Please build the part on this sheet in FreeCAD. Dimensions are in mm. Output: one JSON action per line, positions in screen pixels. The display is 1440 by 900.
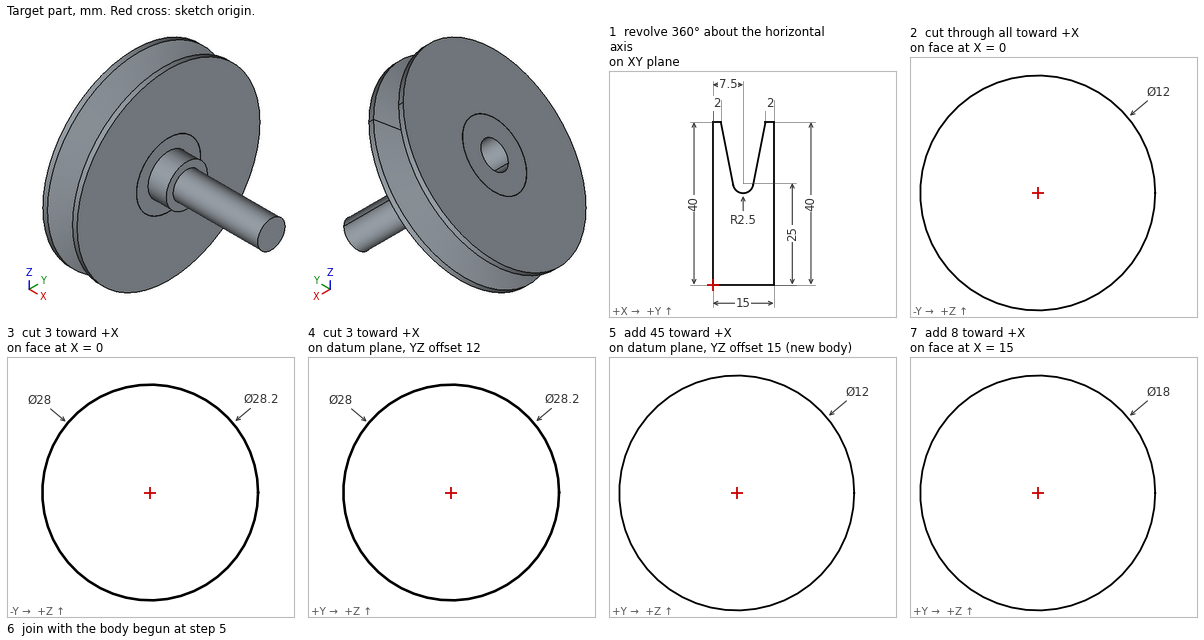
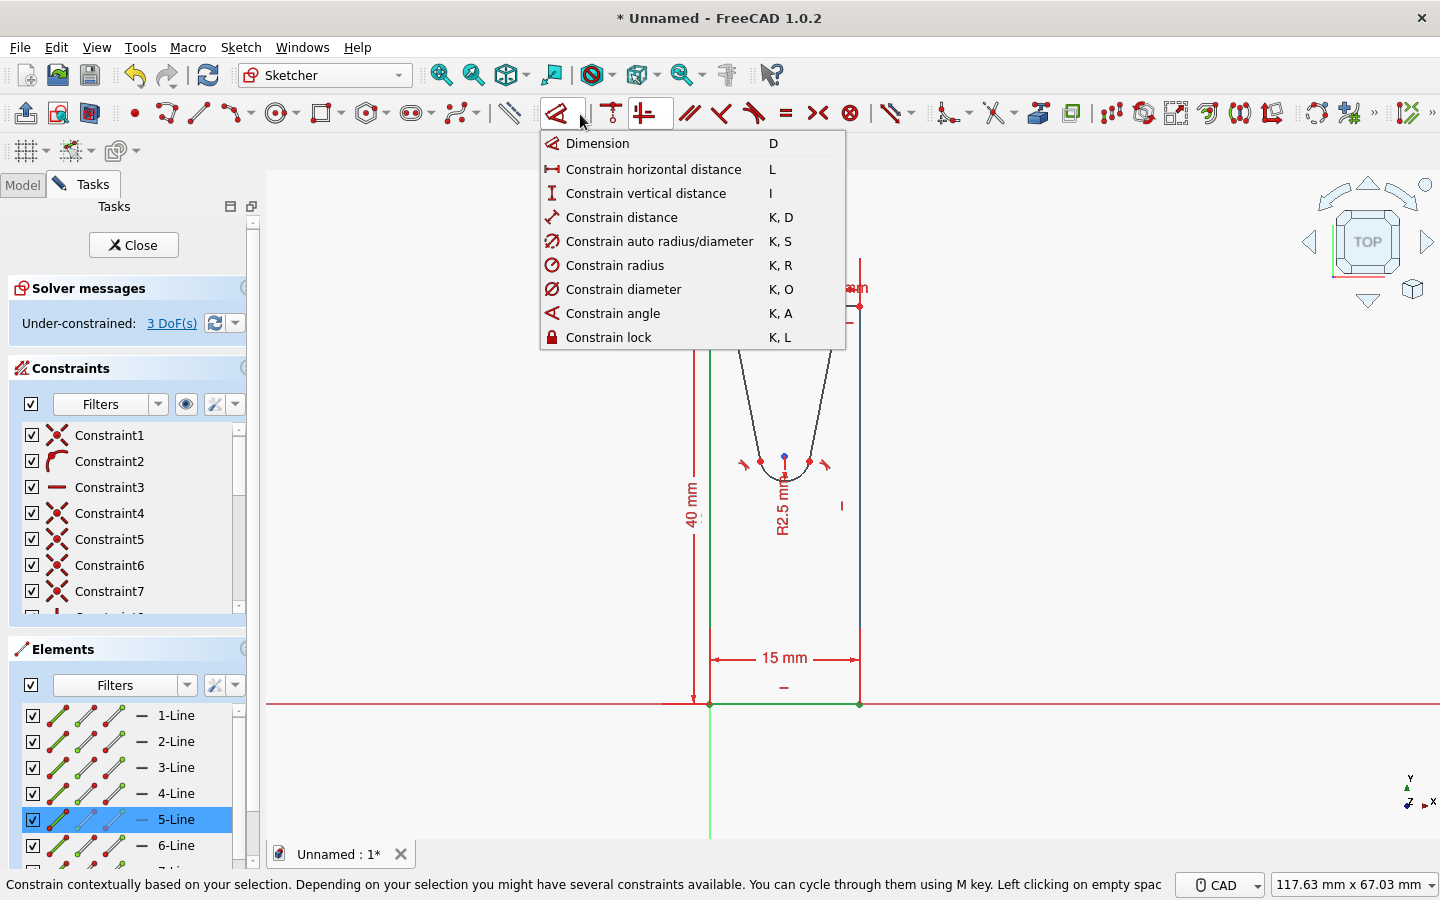
{"action": "left_click", "coordinate": [693, 193]}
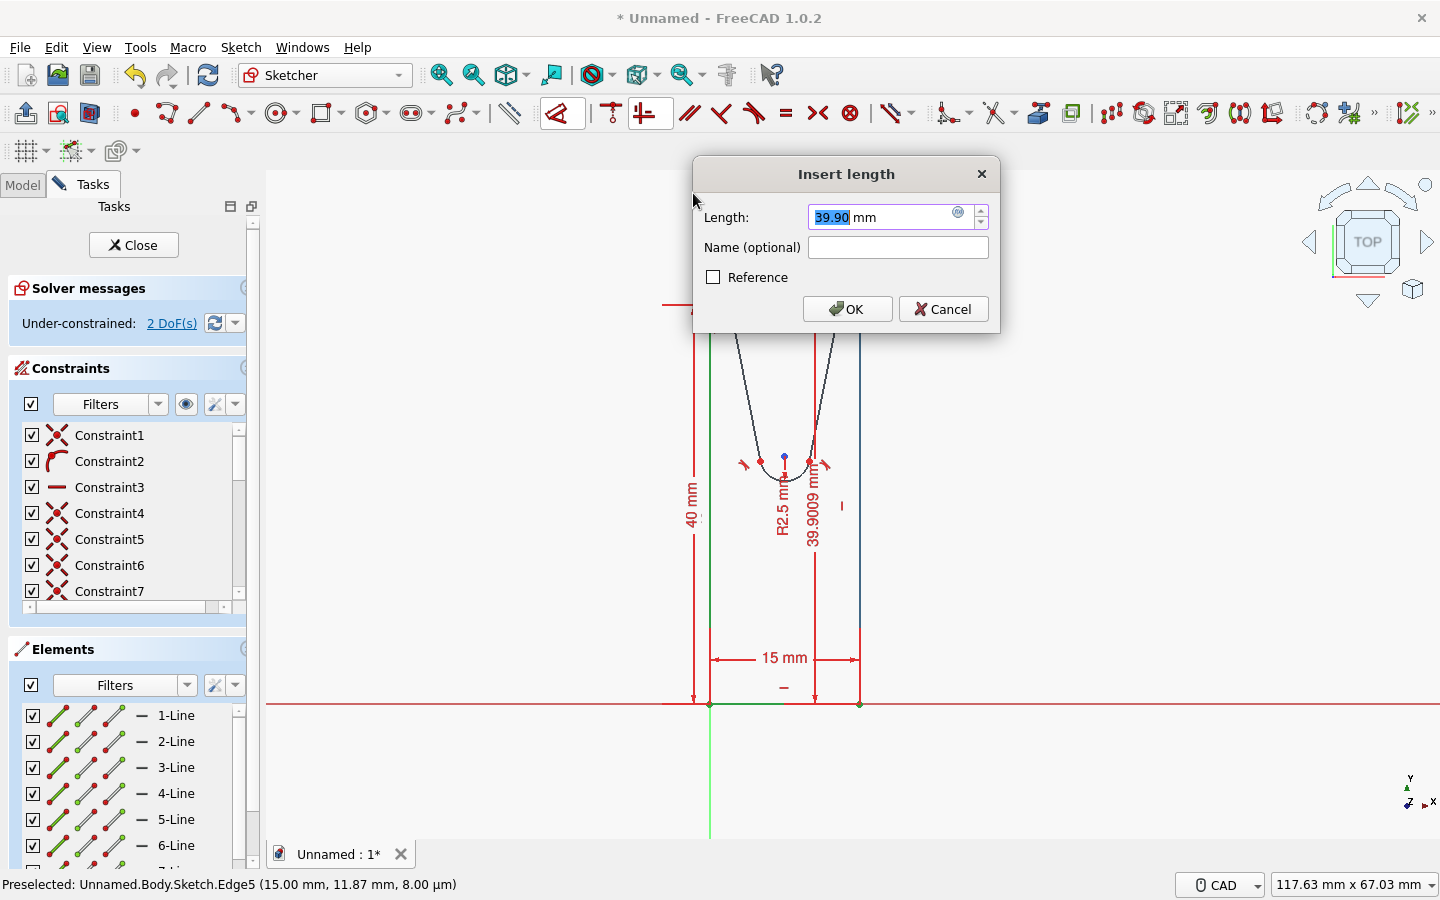
{"action": "type", "text": "40"}
{"action": "key", "text": "Return"}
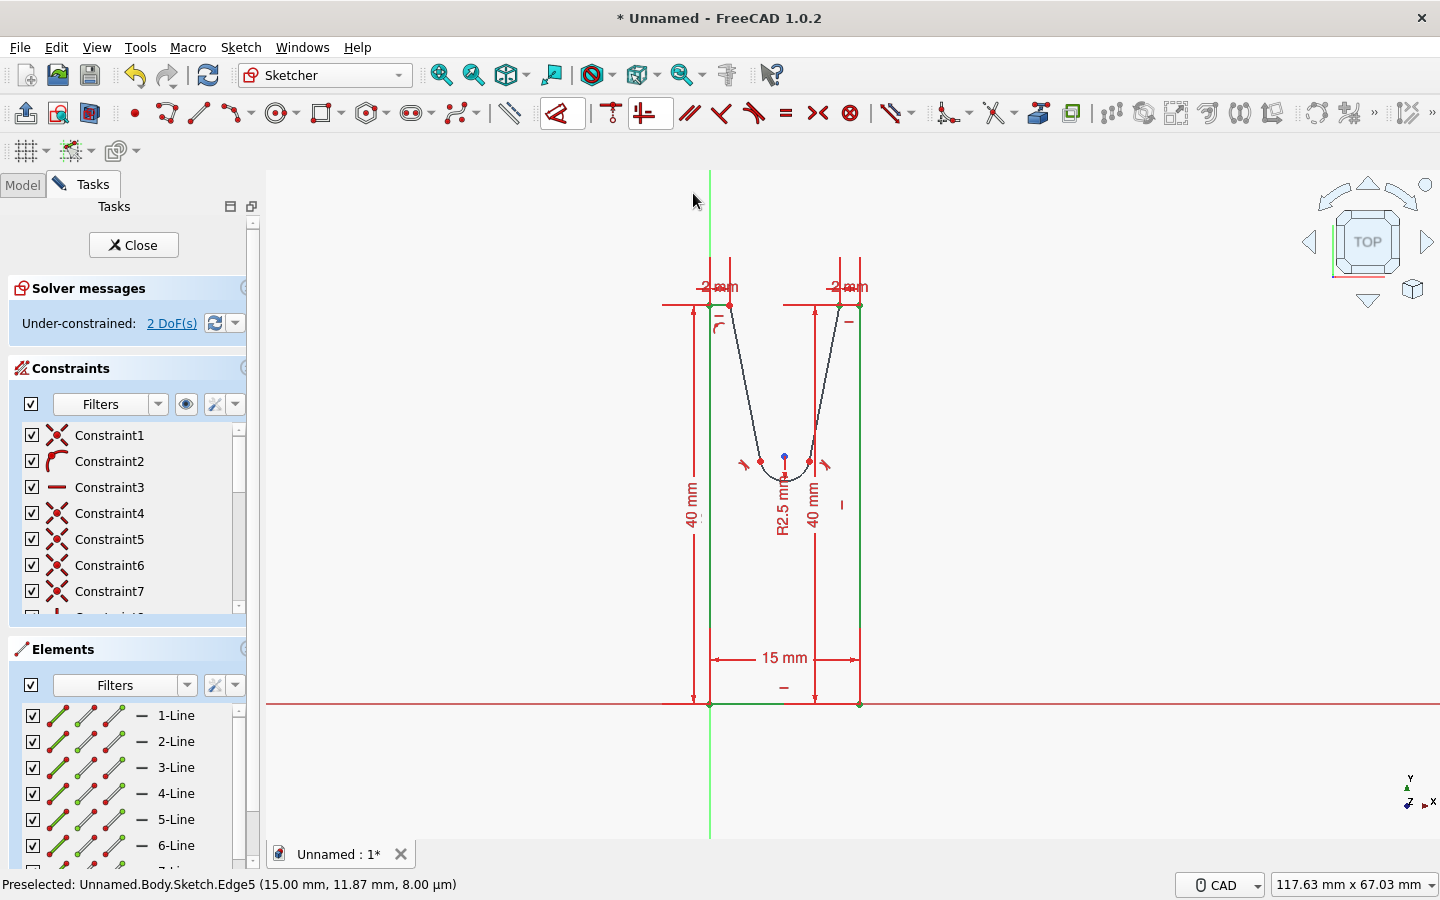
{"action": "left_click", "coordinate": [785, 456]}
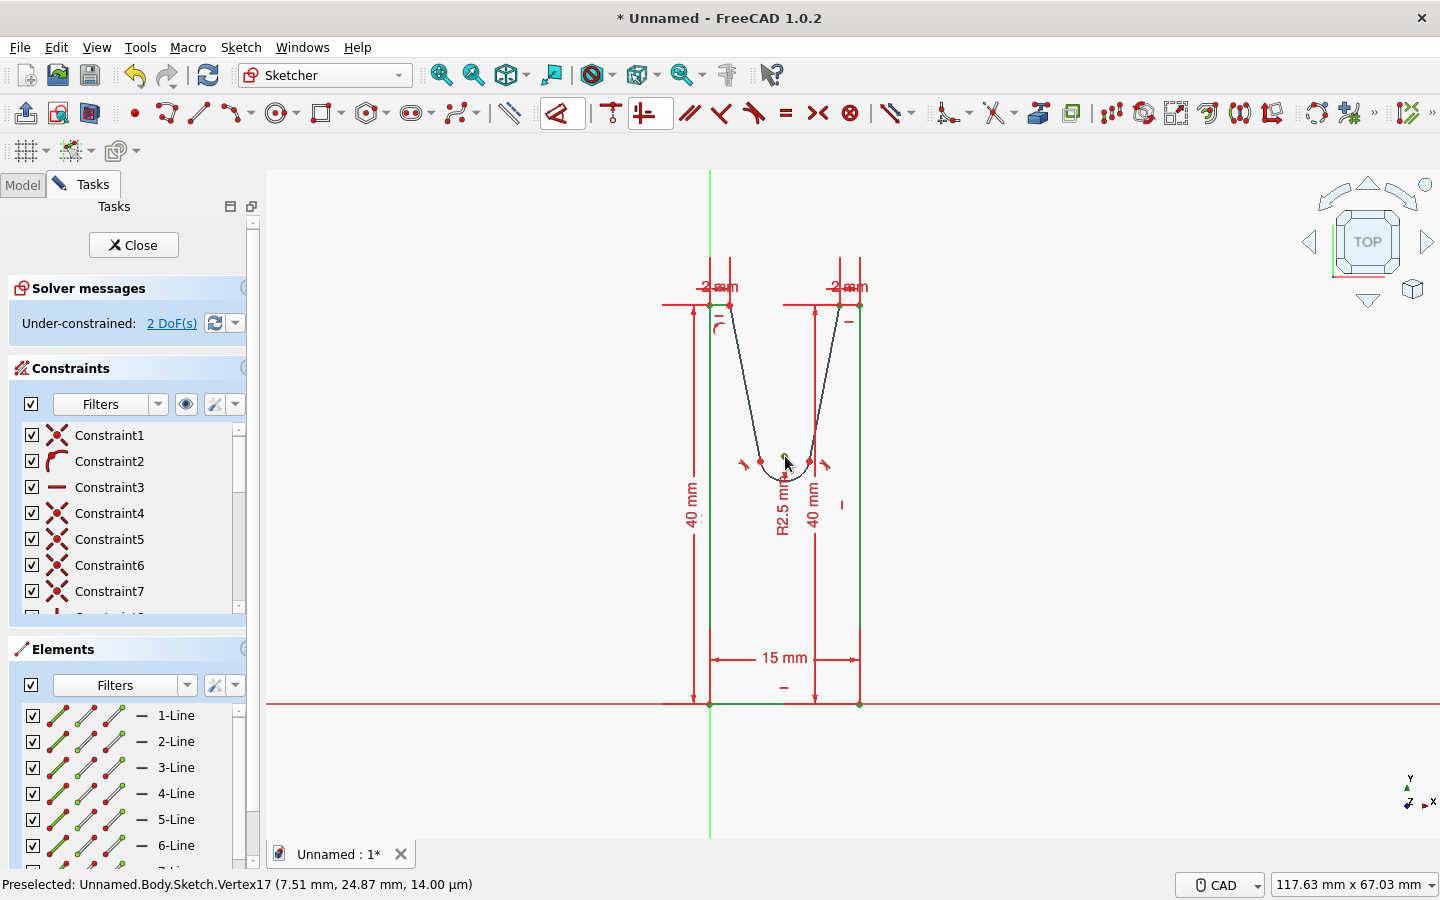
{"action": "left_click", "coordinate": [580, 114]}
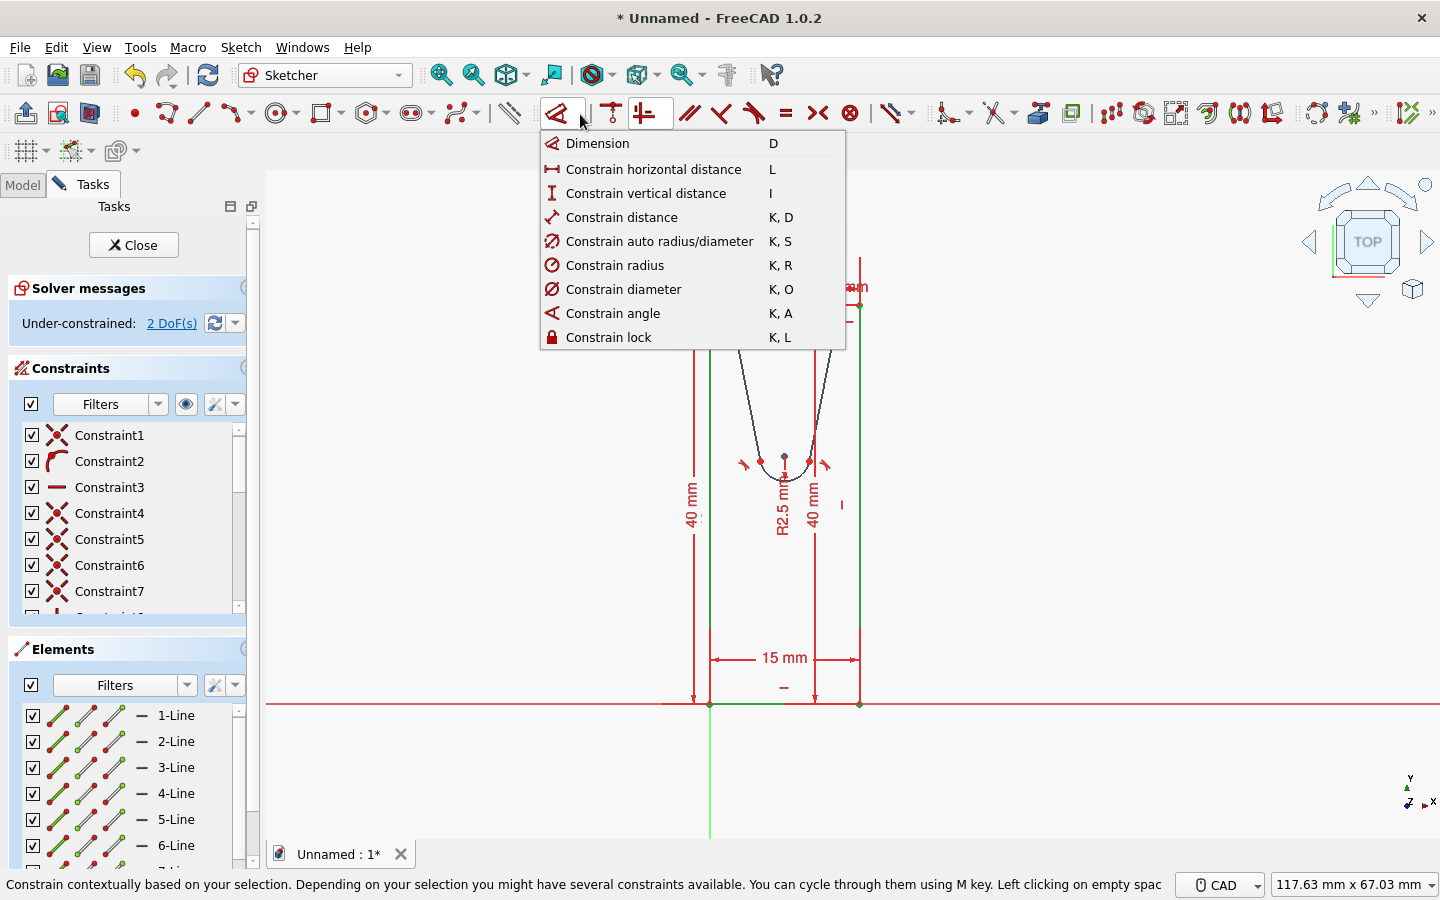
{"action": "left_click", "coordinate": [693, 193]}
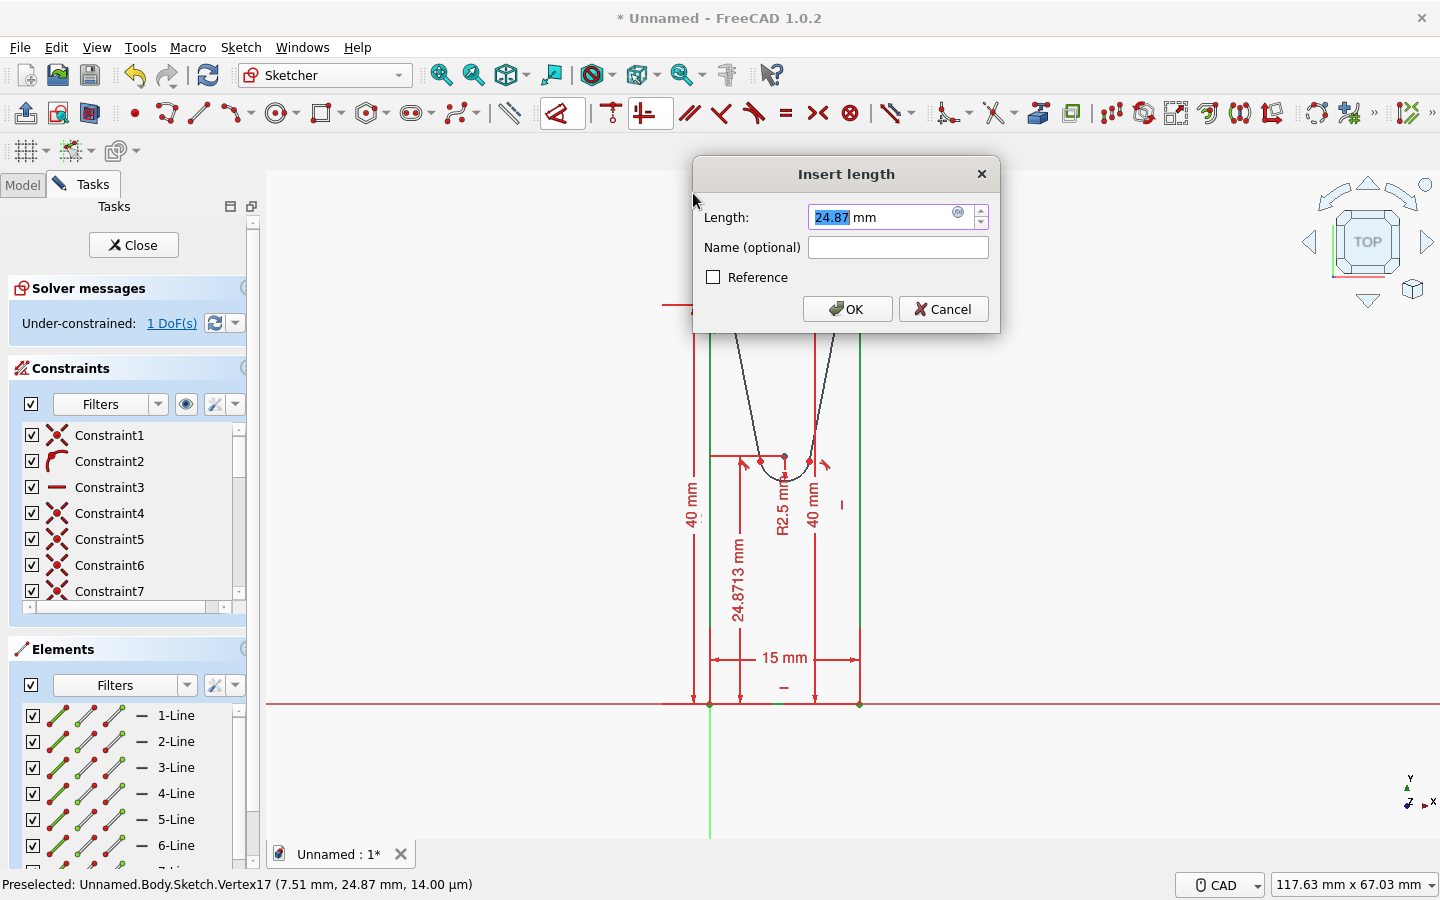
{"action": "type", "text": "25"}
{"action": "key", "text": "Return"}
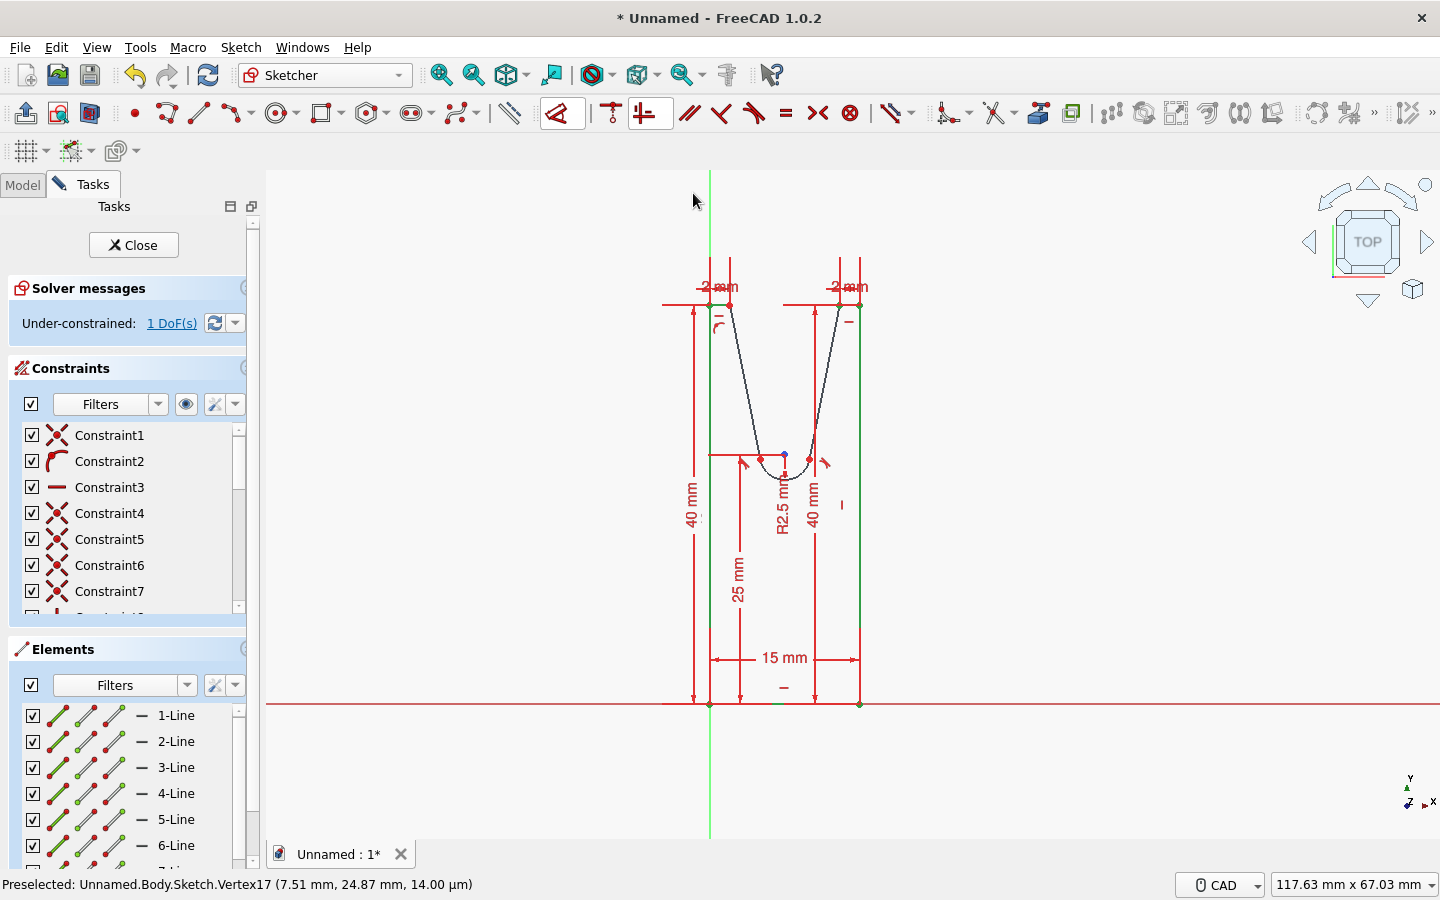
{"action": "left_click", "coordinate": [785, 455]}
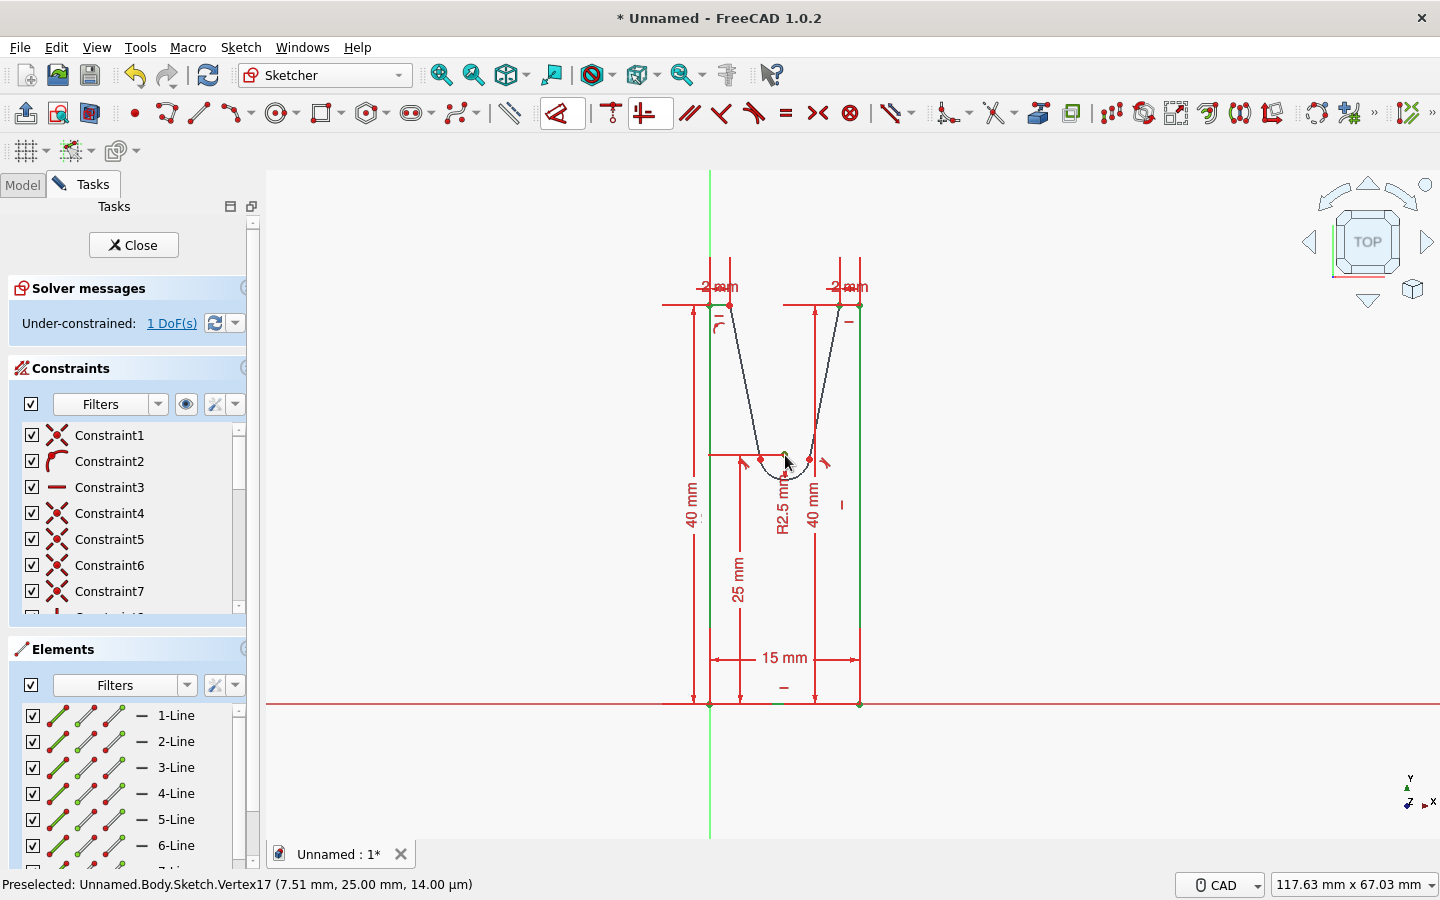
{"action": "key", "text": "l"}